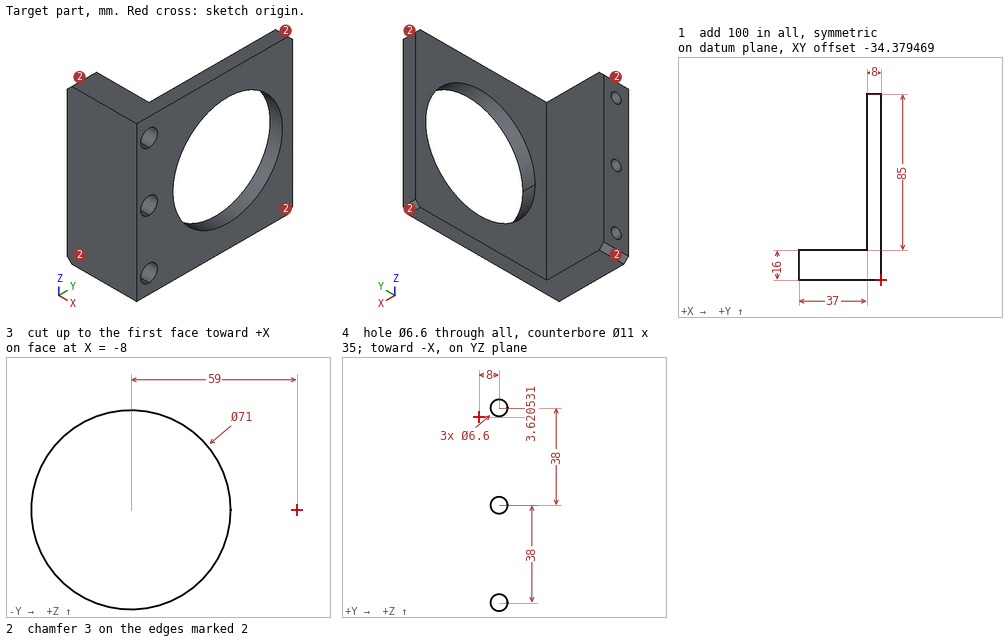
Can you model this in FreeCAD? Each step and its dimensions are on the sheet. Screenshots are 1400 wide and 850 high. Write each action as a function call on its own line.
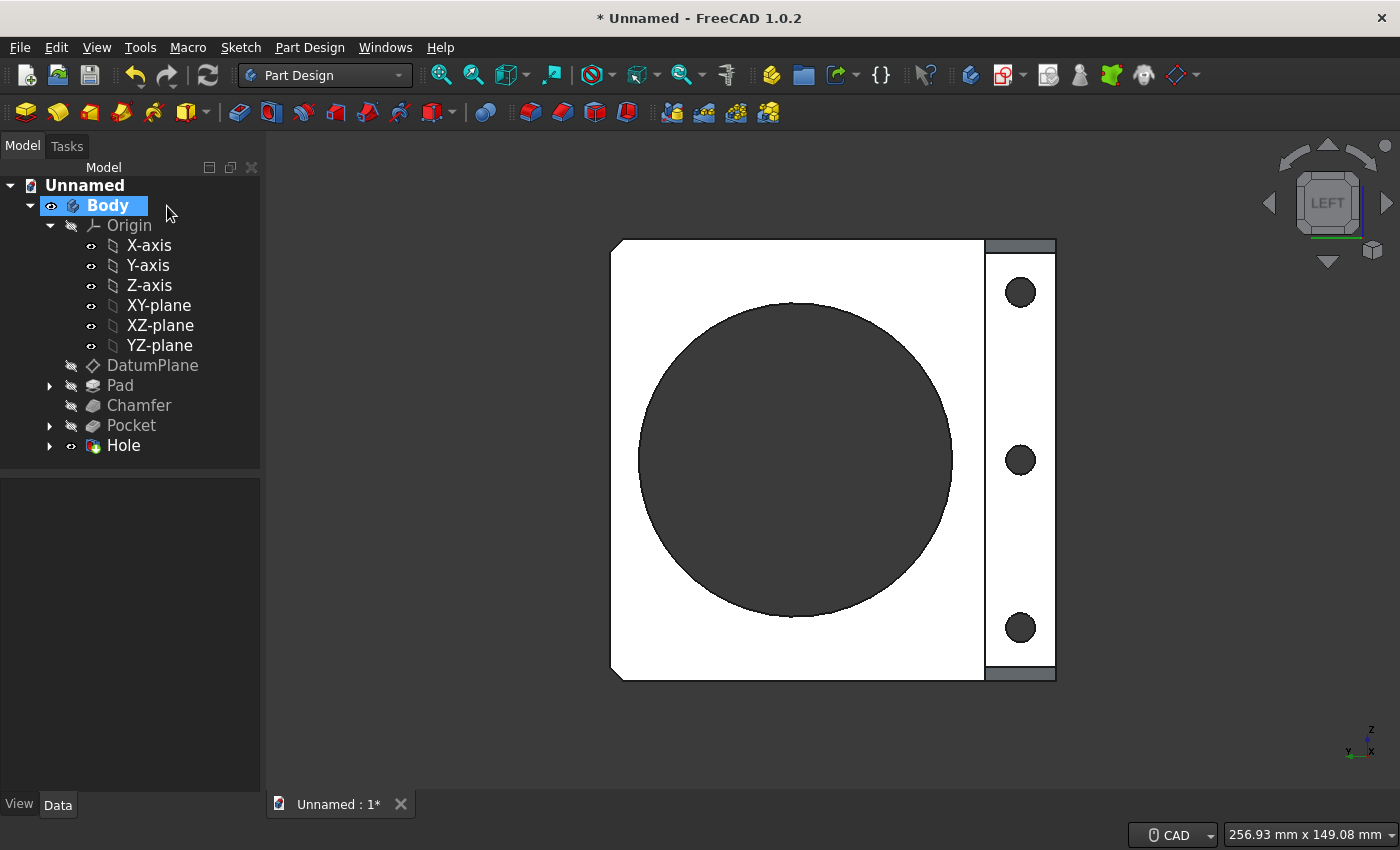
key(0)